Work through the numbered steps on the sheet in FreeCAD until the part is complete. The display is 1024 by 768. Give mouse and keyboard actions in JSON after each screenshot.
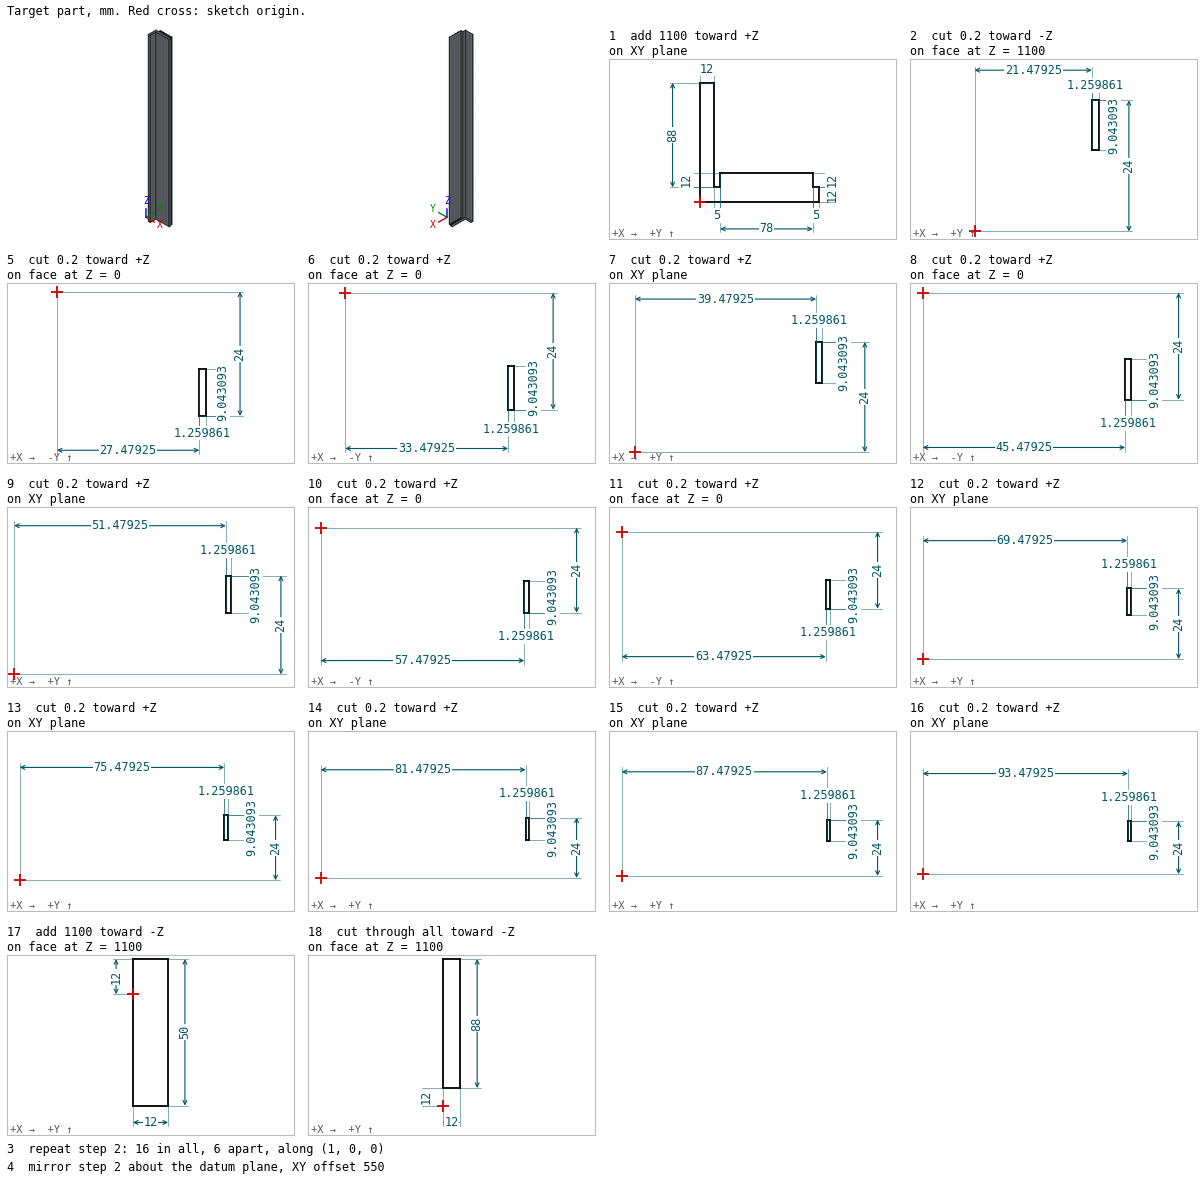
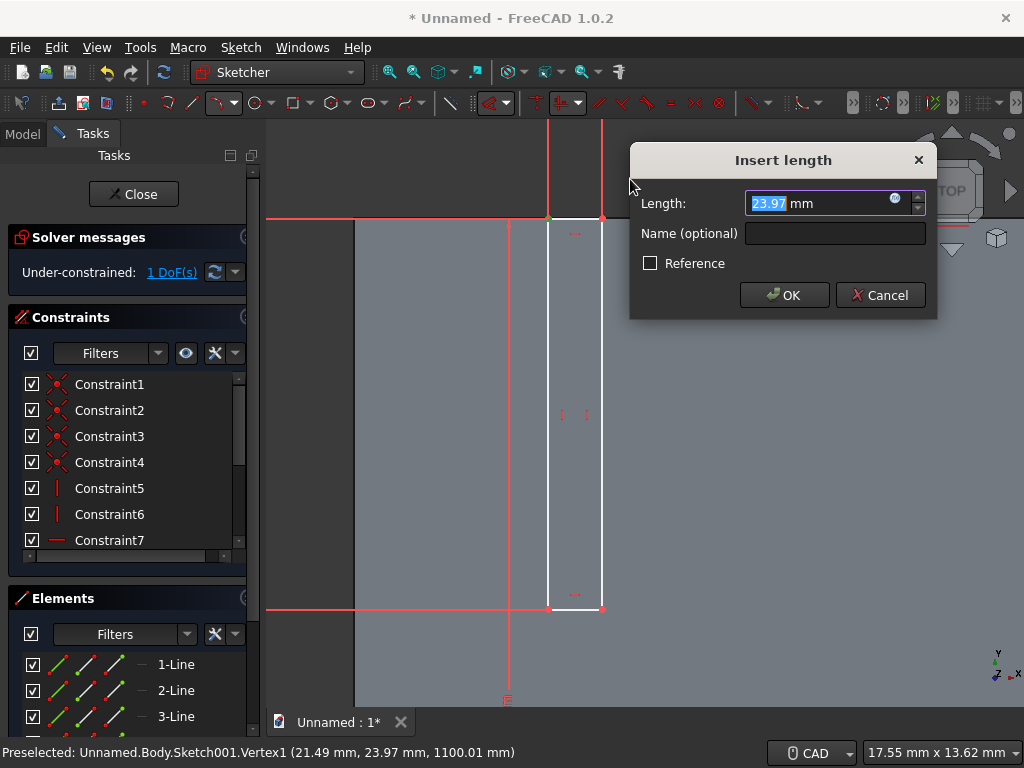
{"action": "type", "text": "24"}
{"action": "key", "text": "Return"}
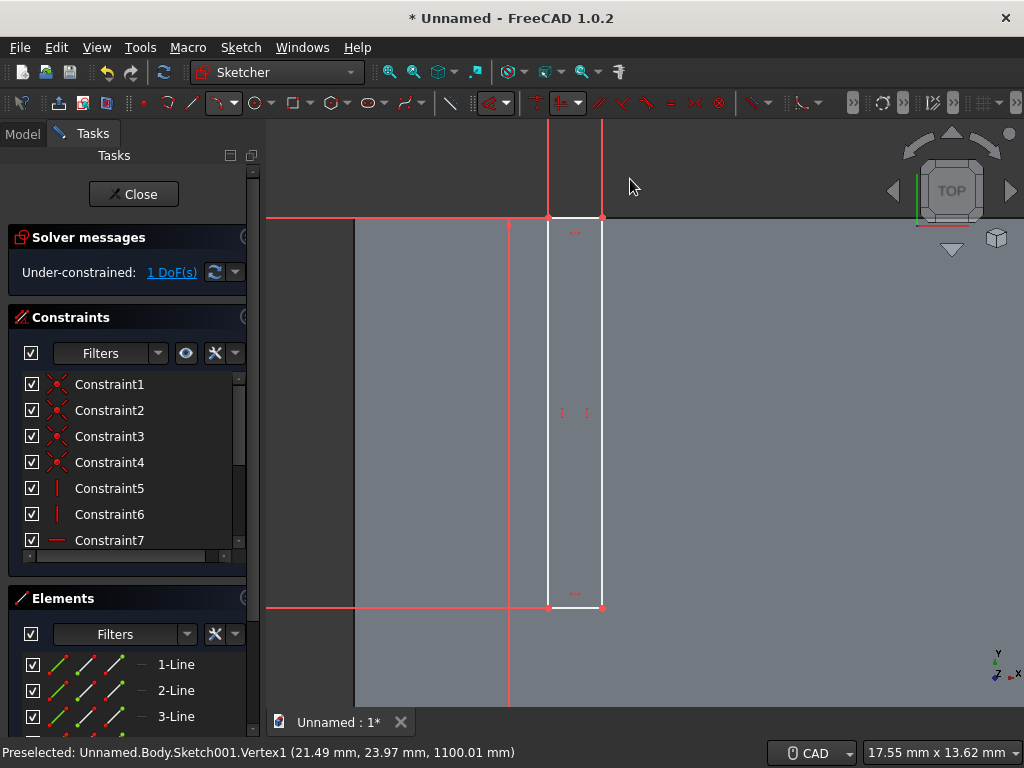
{"action": "left_click", "coordinate": [548, 218]}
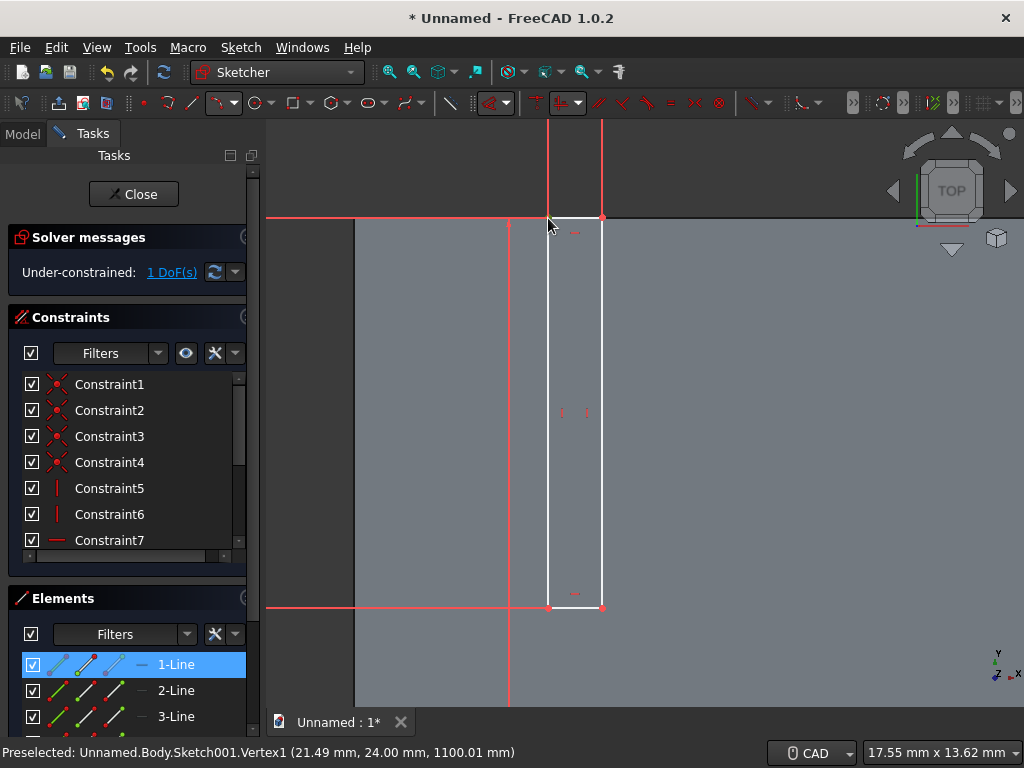
{"action": "key", "text": "l"}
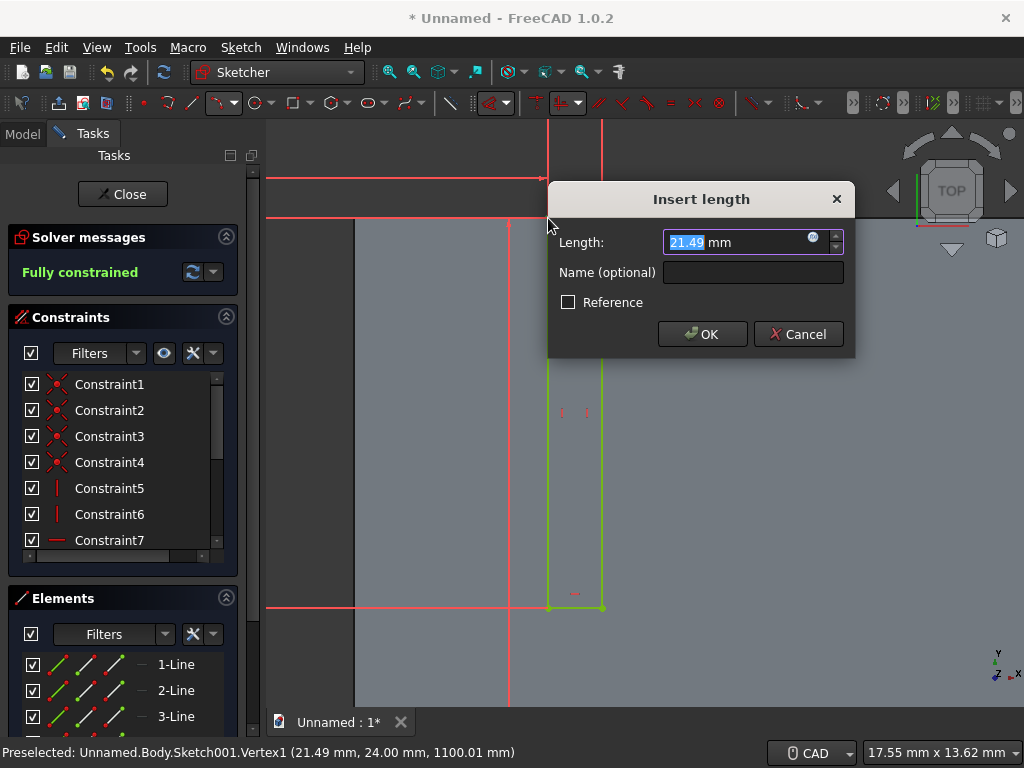
{"action": "type", "text": "21.47925"}
{"action": "key", "text": "Return"}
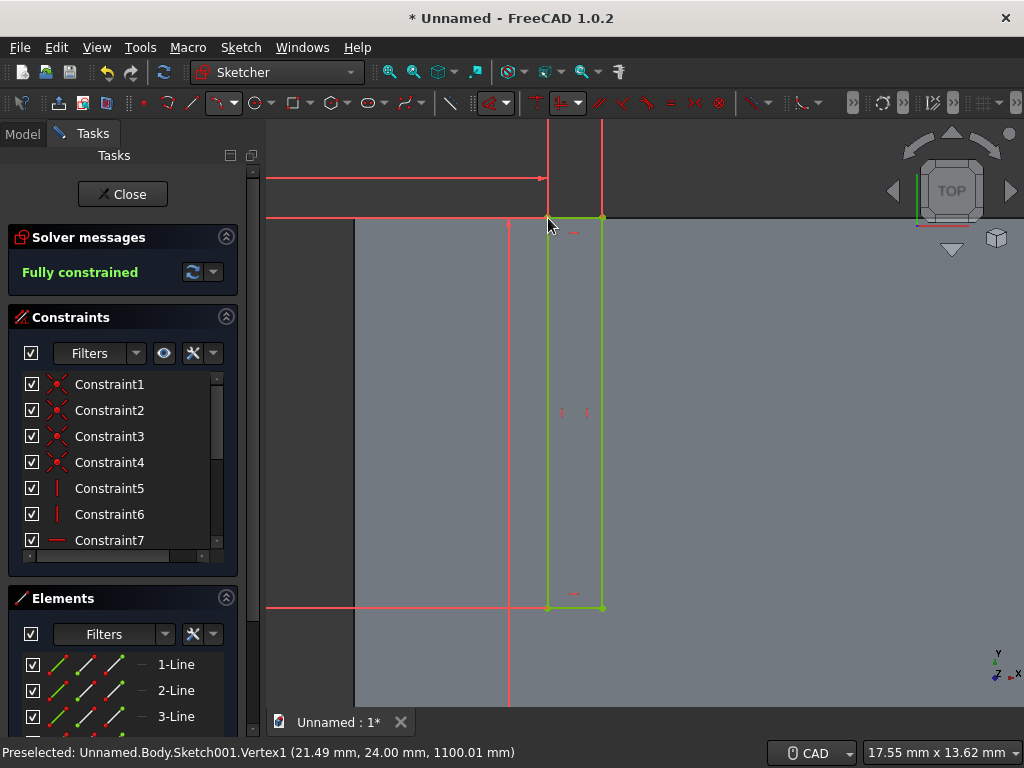
{"action": "left_click", "coordinate": [123, 194]}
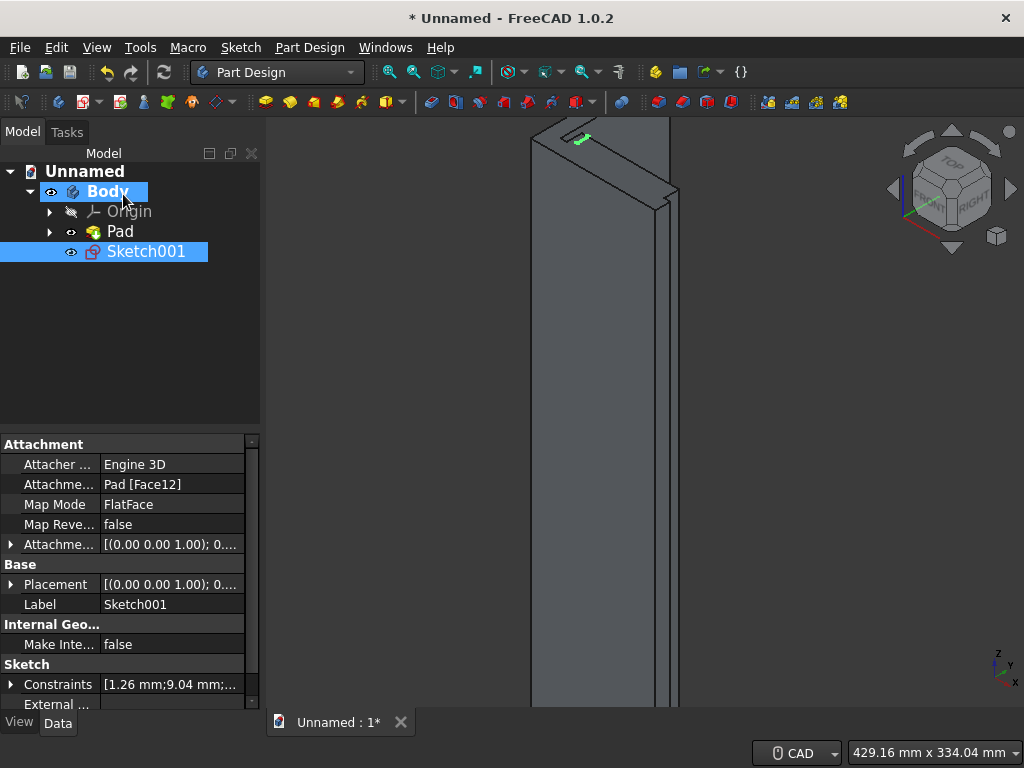
{"action": "left_click", "coordinate": [432, 102]}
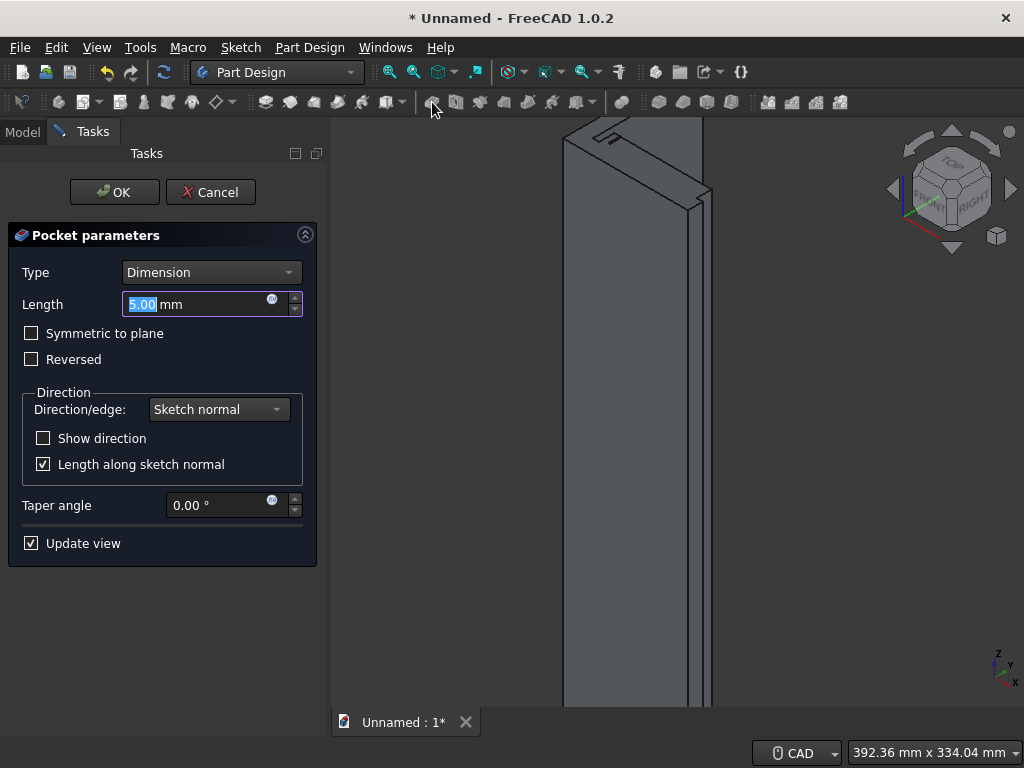
{"action": "type", "text": "0.2"}
{"action": "key", "text": "Tab"}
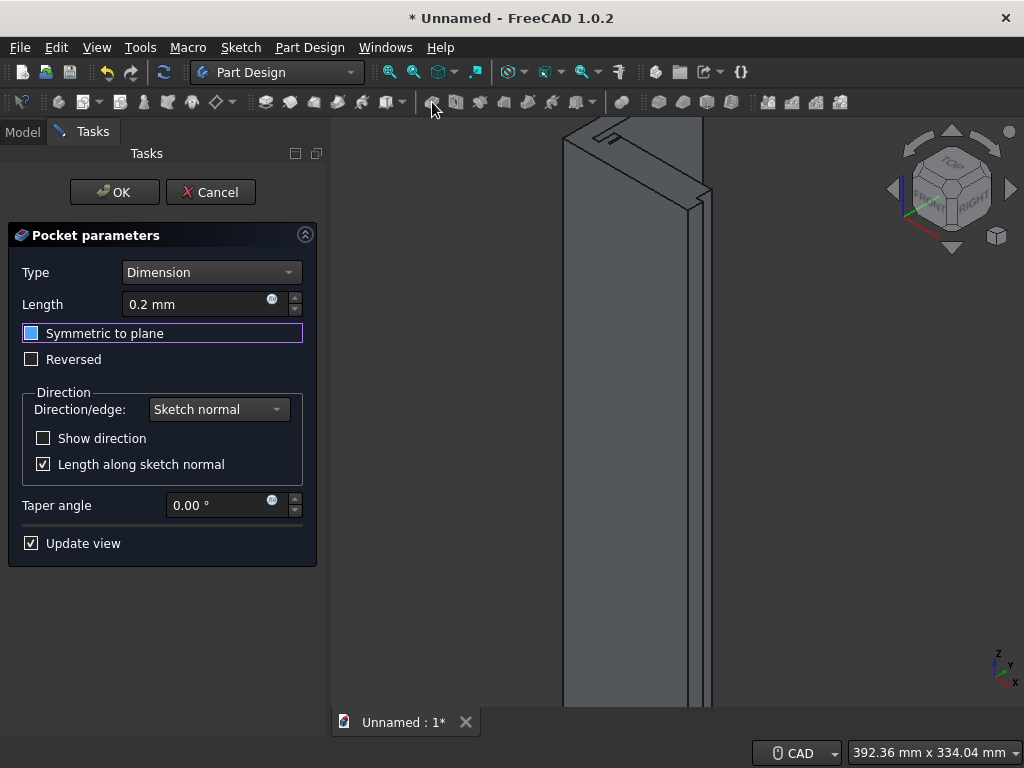
{"action": "left_click", "coordinate": [115, 192]}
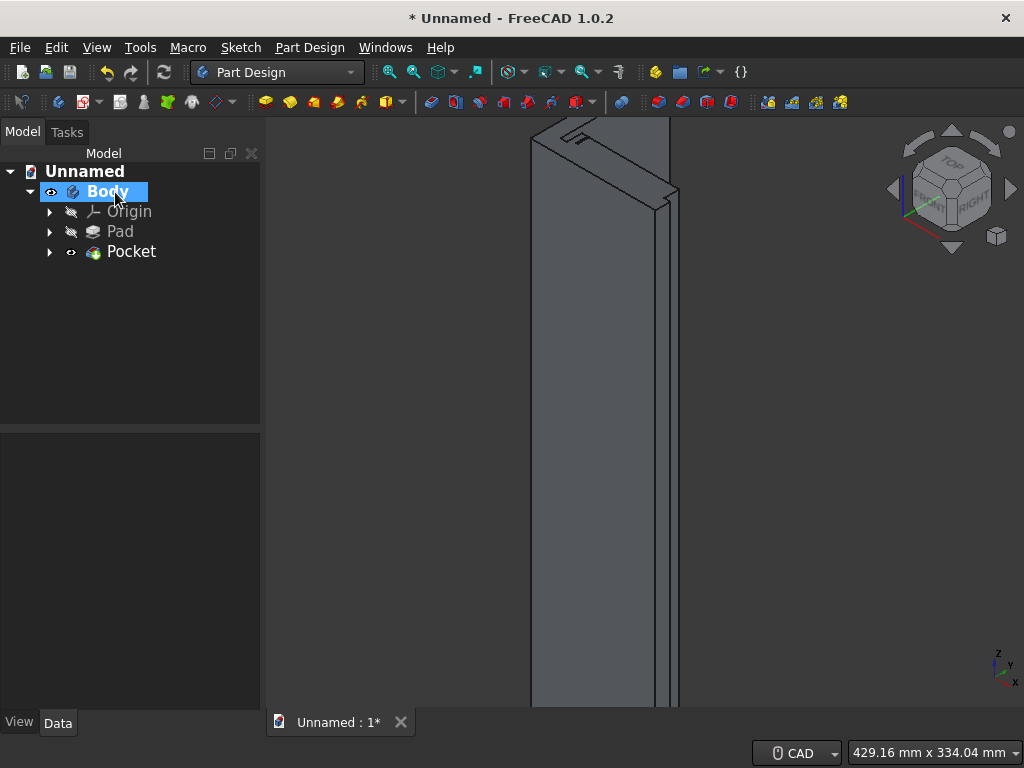
{"action": "key", "text": "v f"}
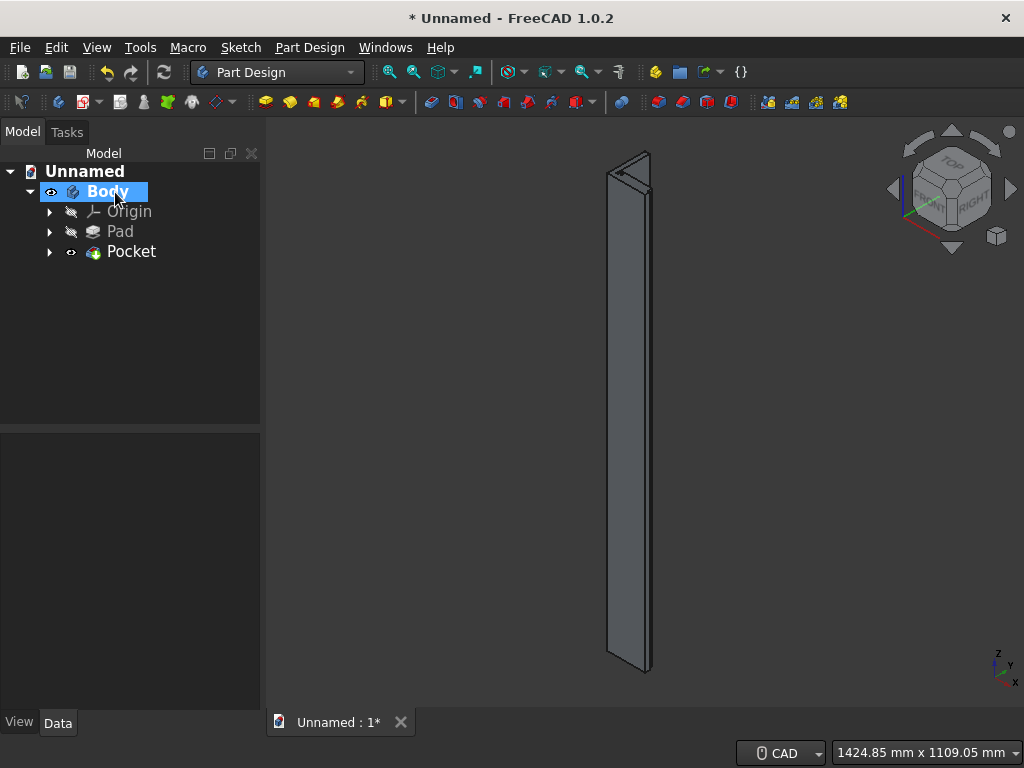
{"action": "left_click", "coordinate": [116, 252]}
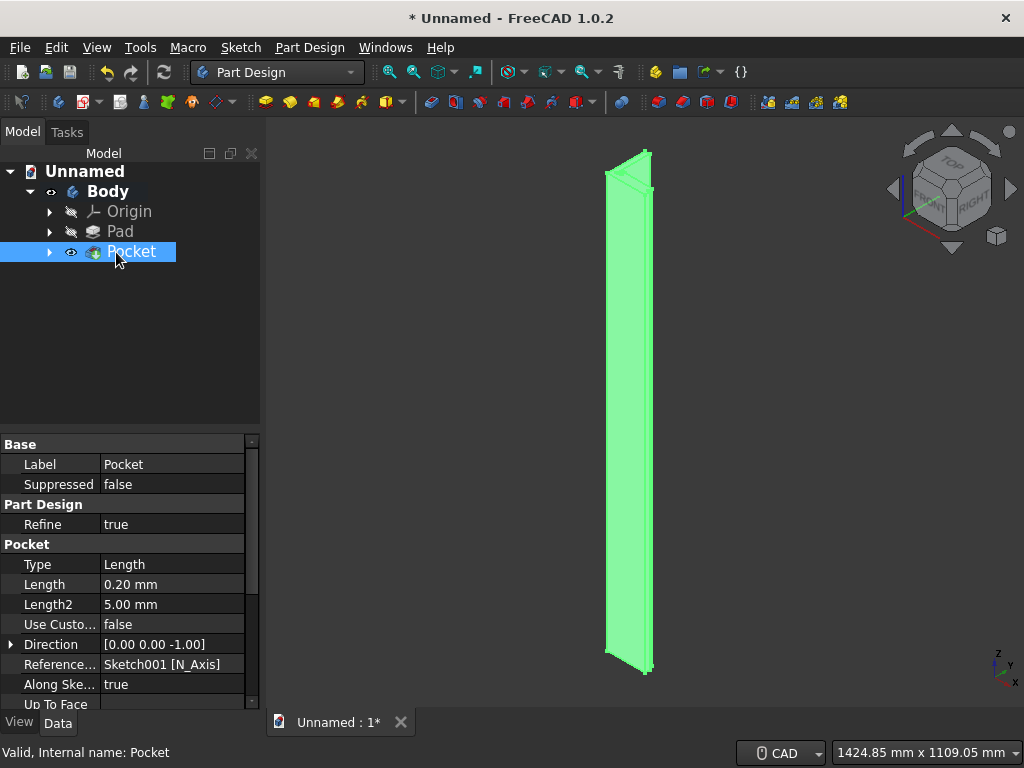
{"action": "left_click", "coordinate": [792, 102]}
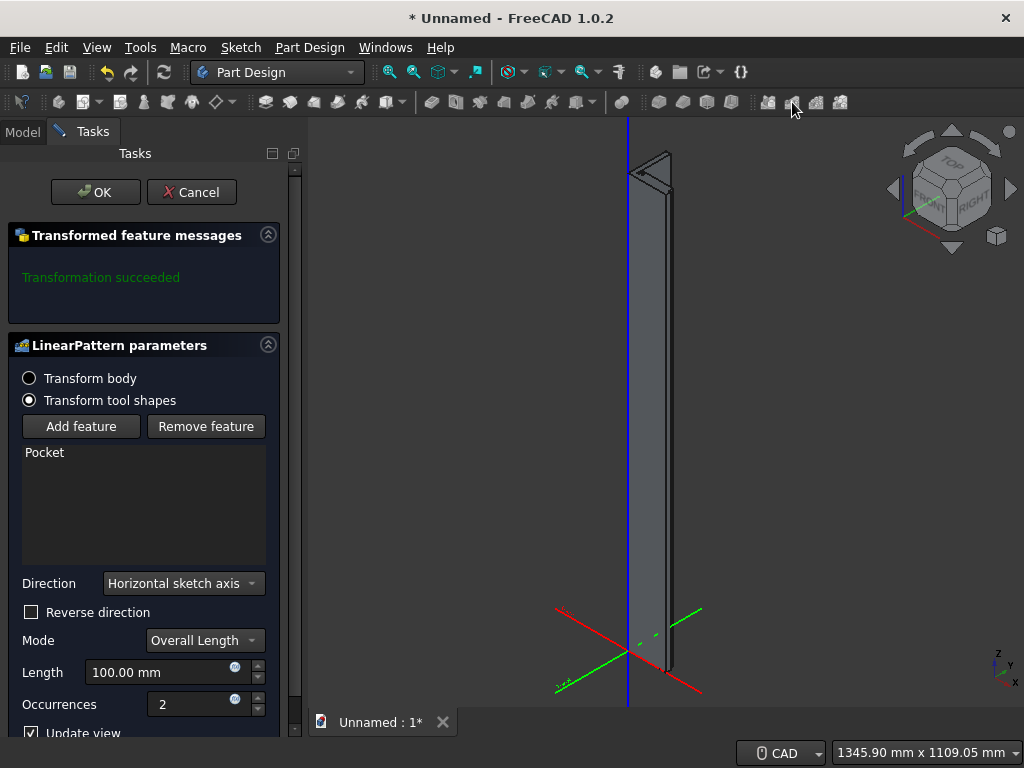
{"action": "left_click", "coordinate": [184, 584]}